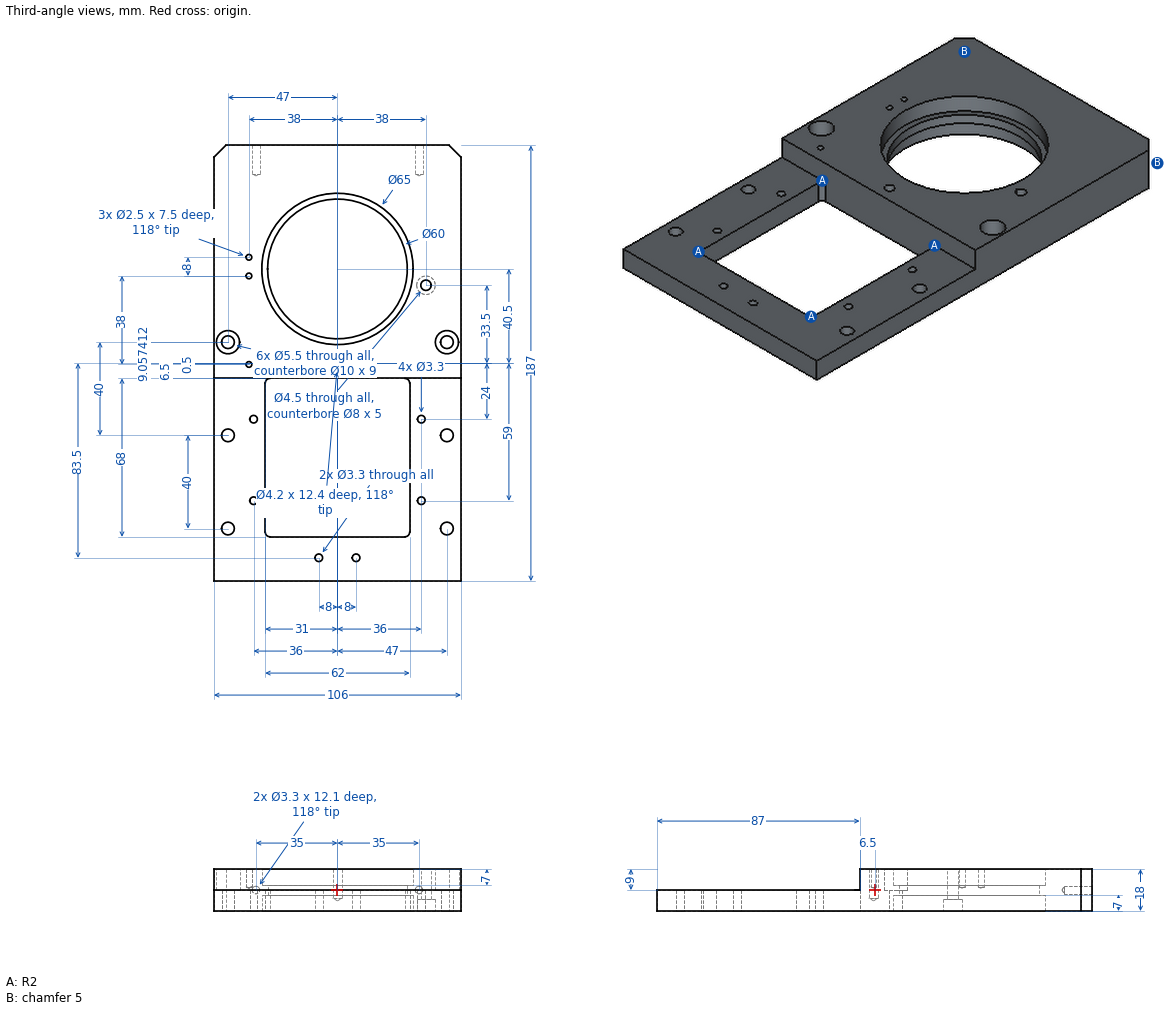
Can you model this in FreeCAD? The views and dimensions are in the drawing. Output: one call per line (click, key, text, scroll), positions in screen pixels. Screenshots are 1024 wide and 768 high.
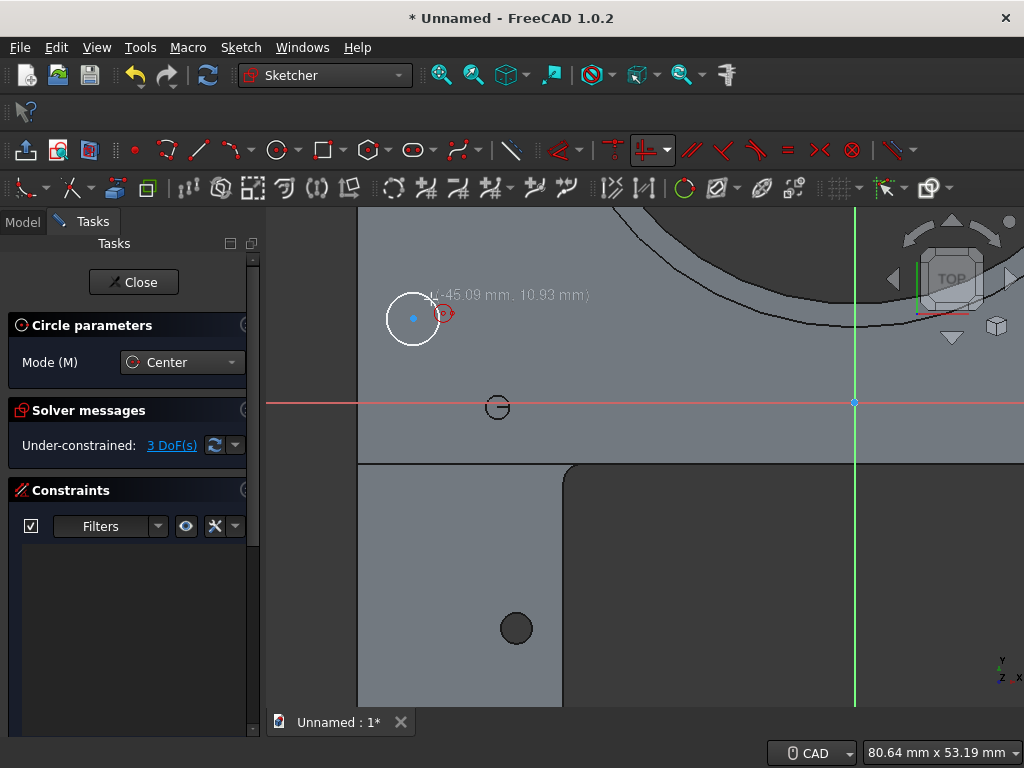
scroll(415, 319, down, 5)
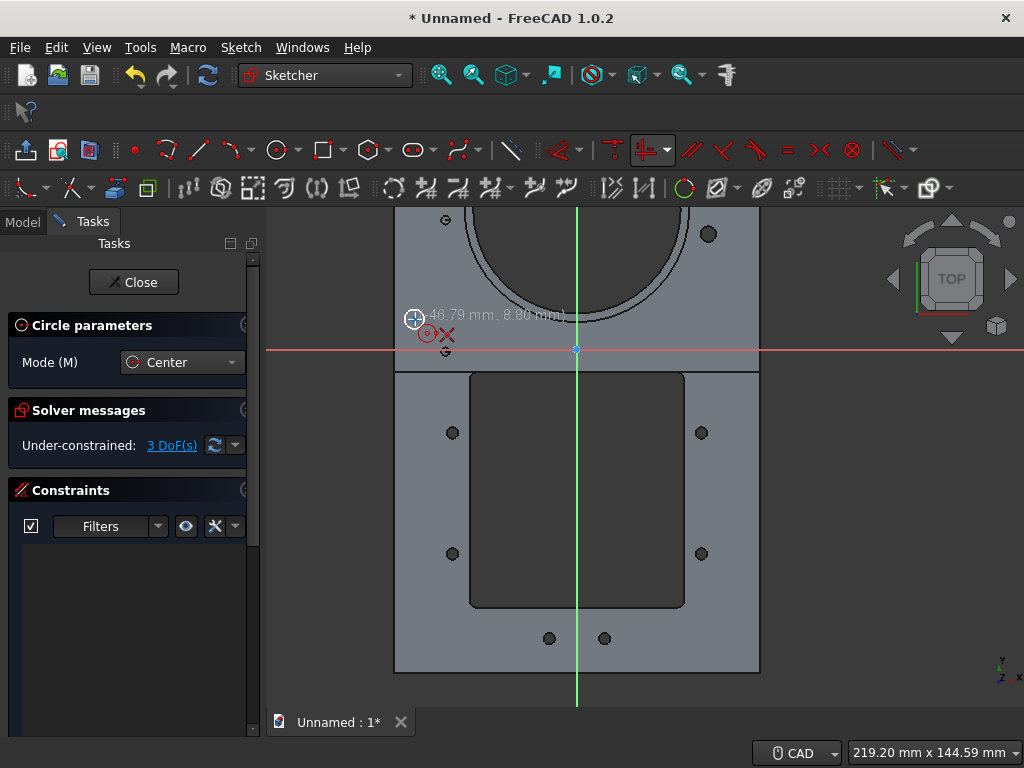
scroll(414, 457, up, 5)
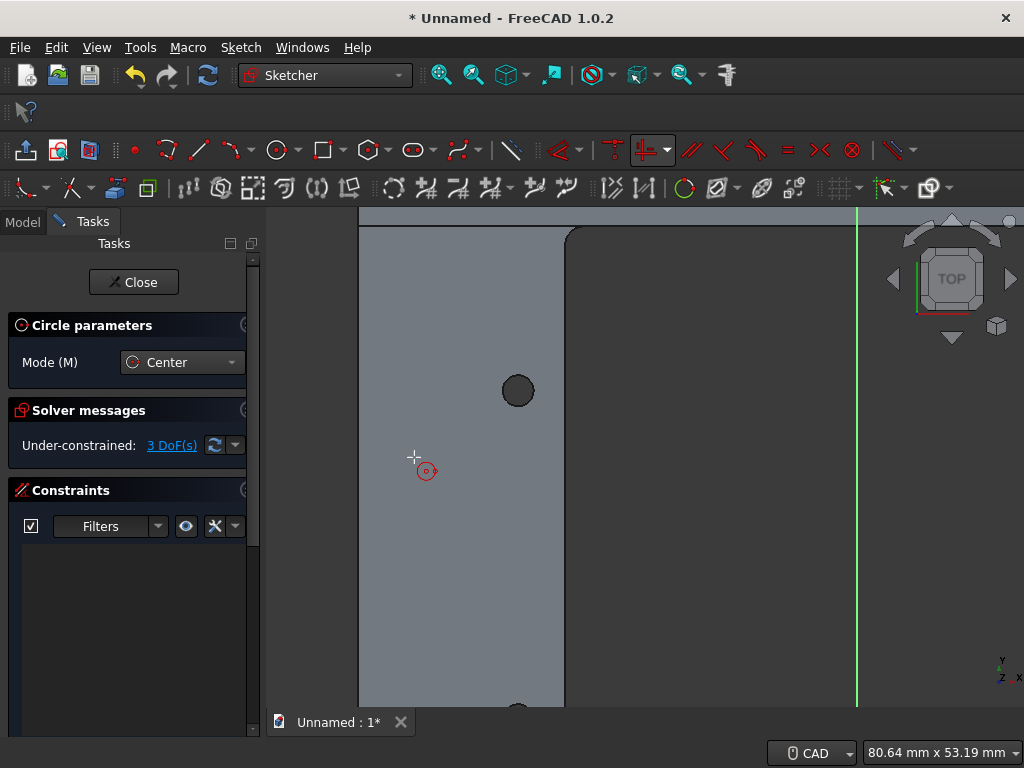
click(415, 456)
click(433, 438)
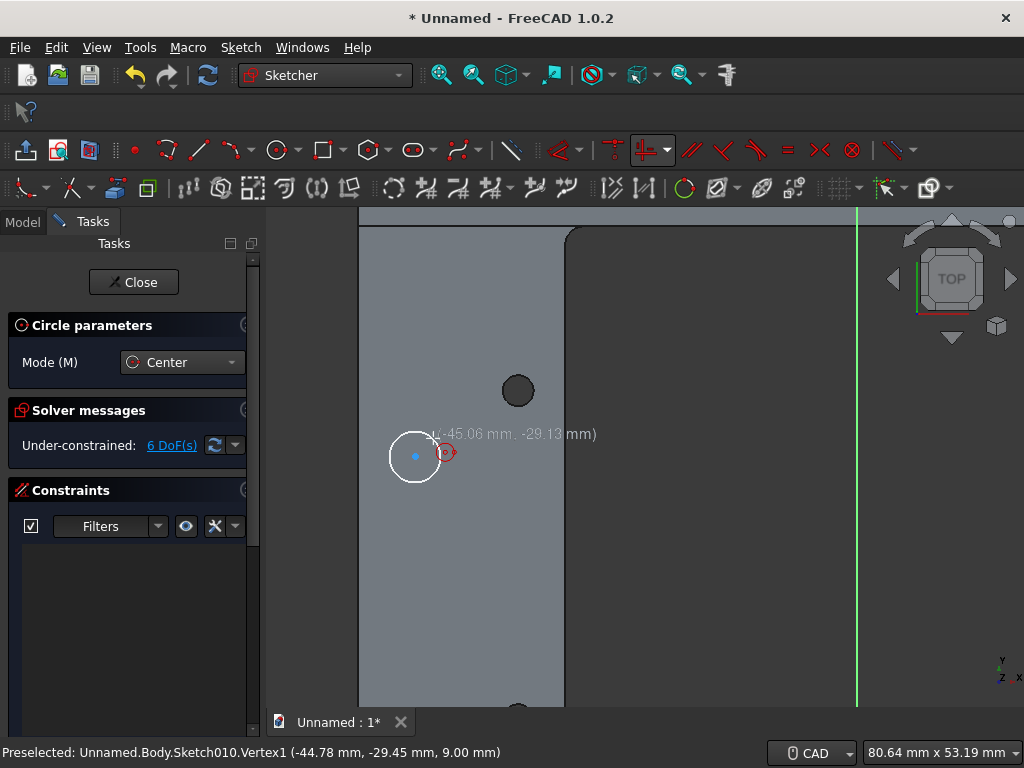
scroll(414, 458, down, 5)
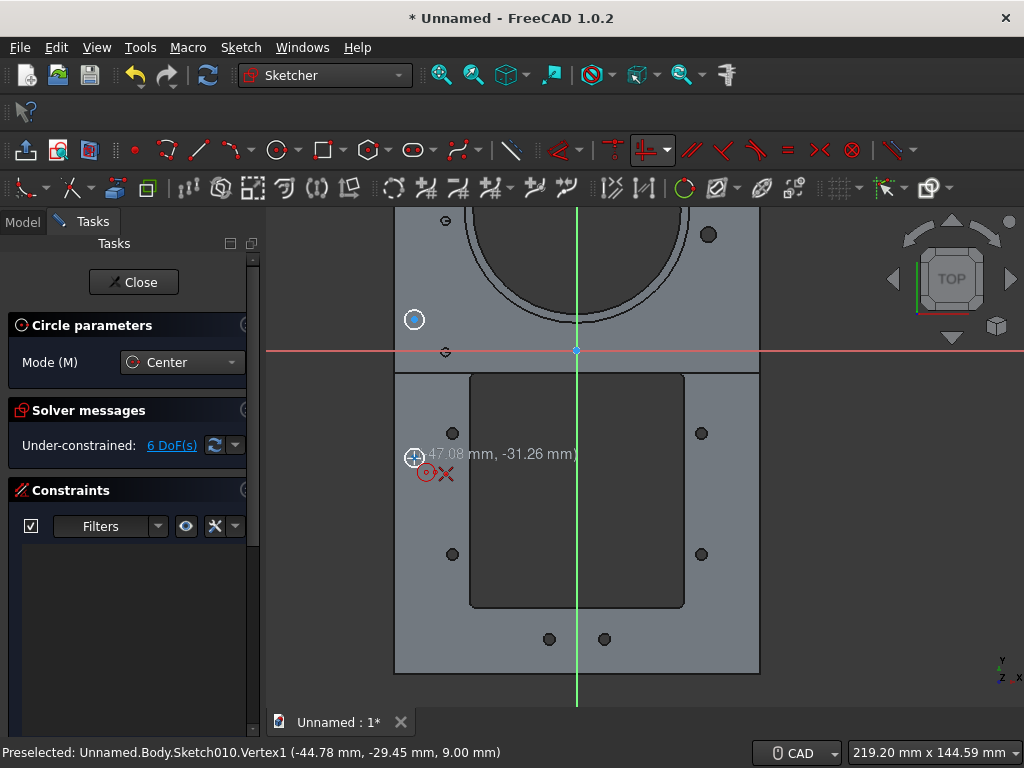
scroll(414, 596, up, 5)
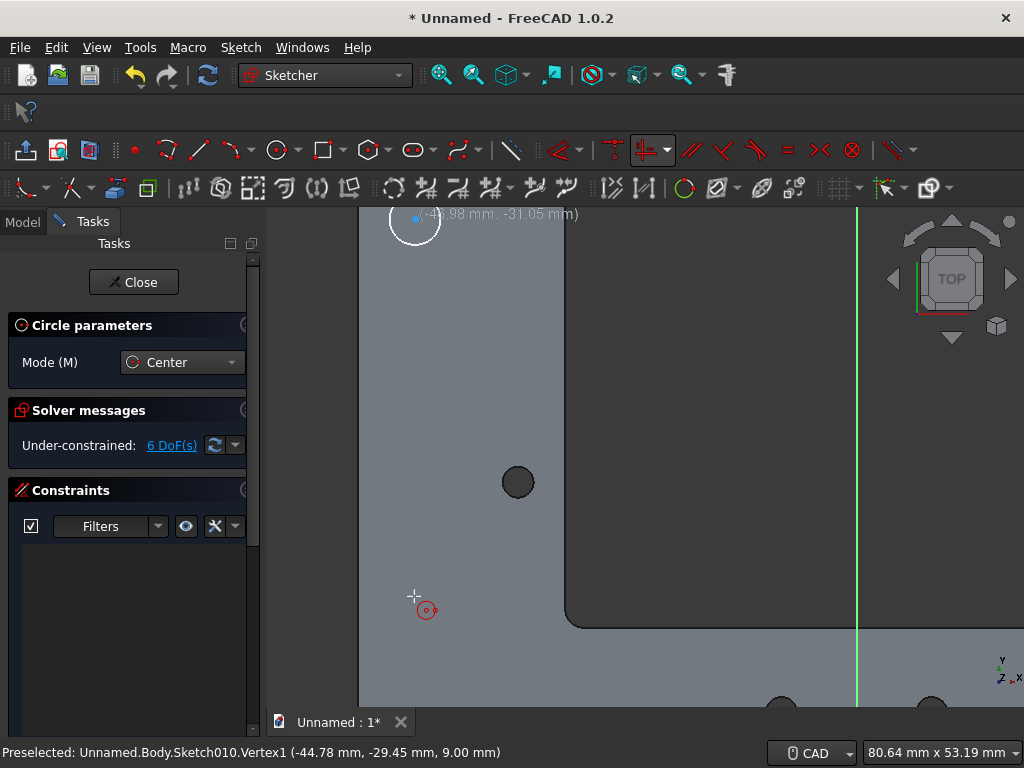
click(415, 594)
click(433, 576)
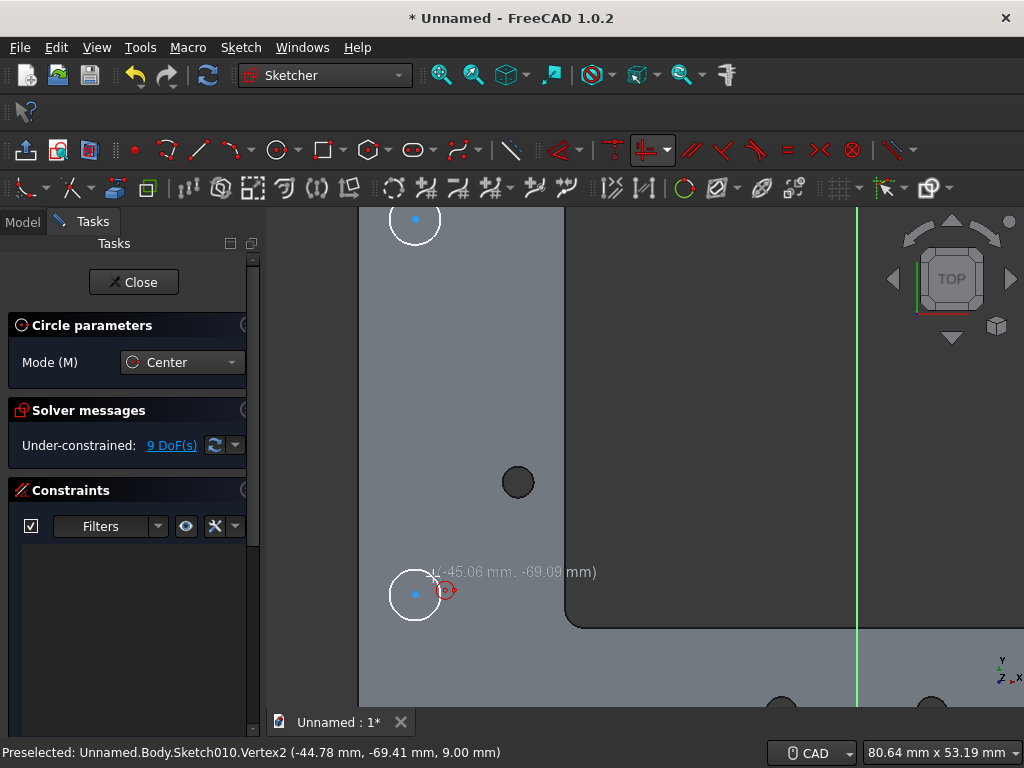
scroll(414, 596, down, 5)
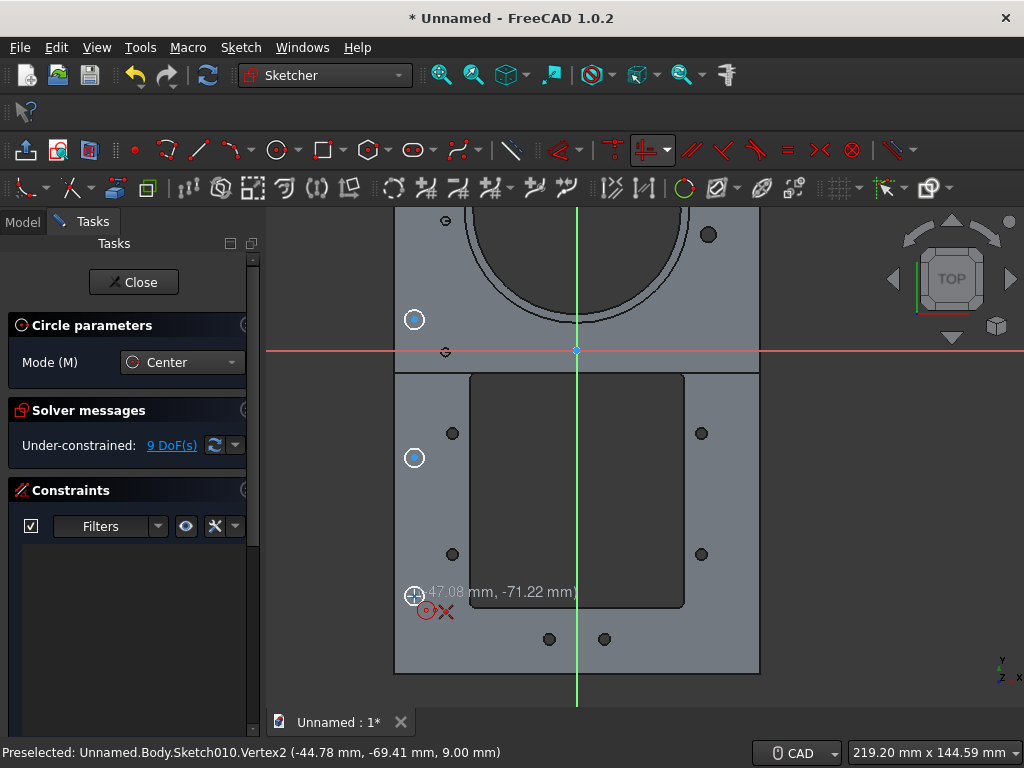
scroll(739, 596, up, 5)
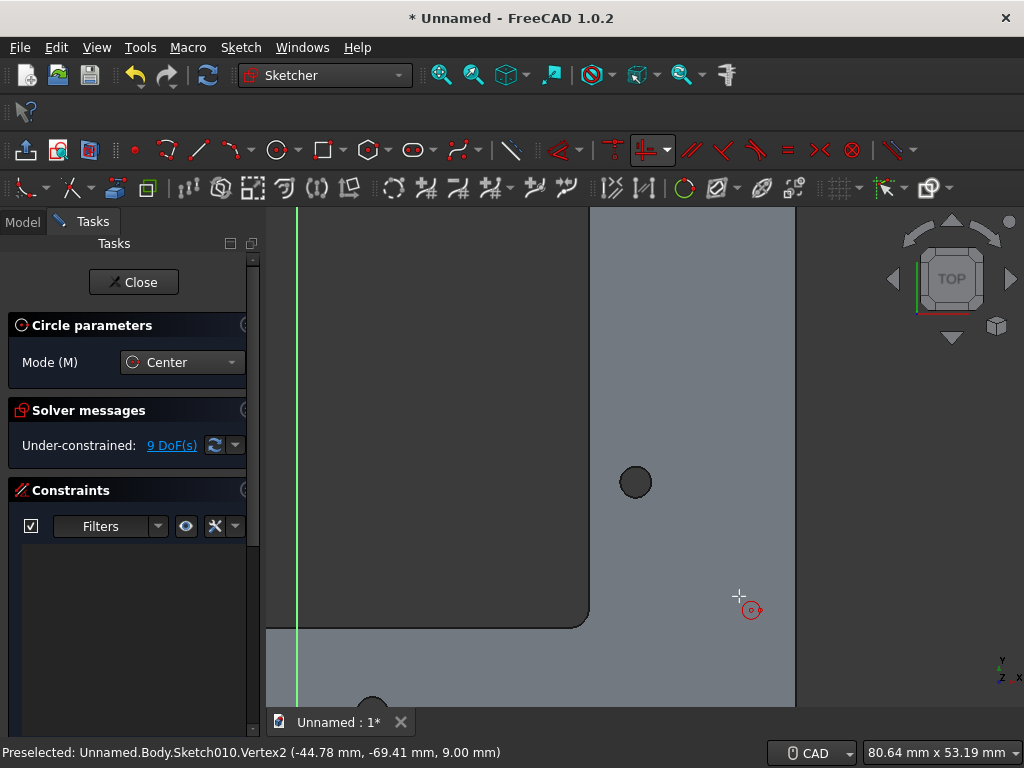
click(739, 594)
click(757, 576)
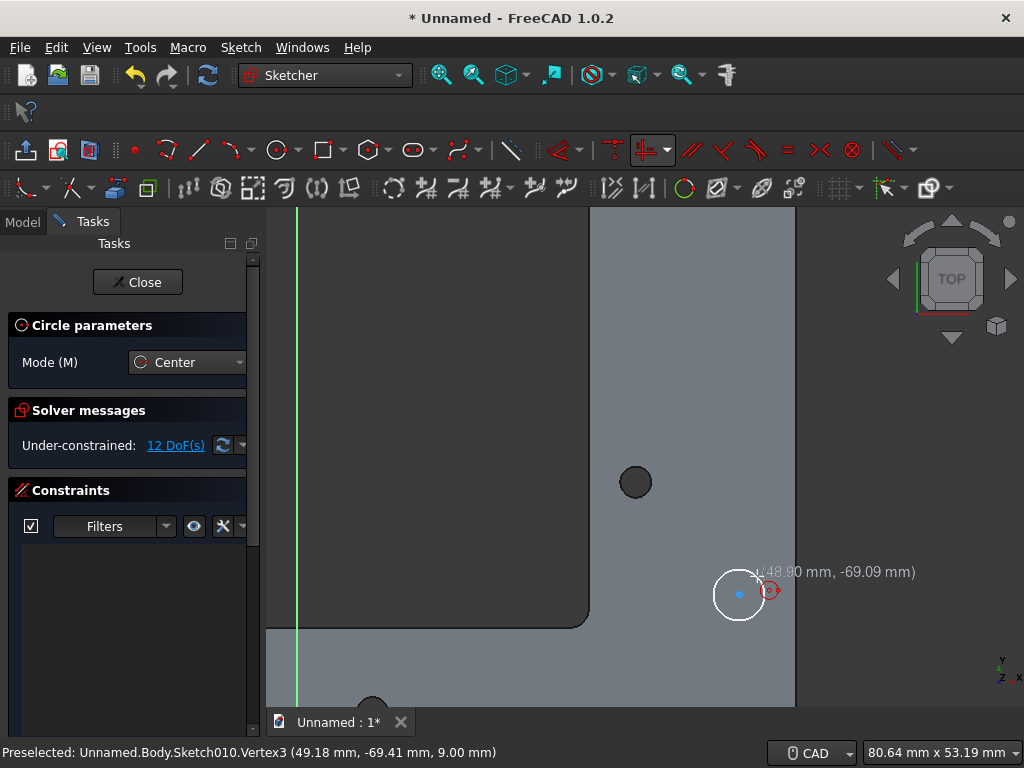
scroll(739, 596, down, 5)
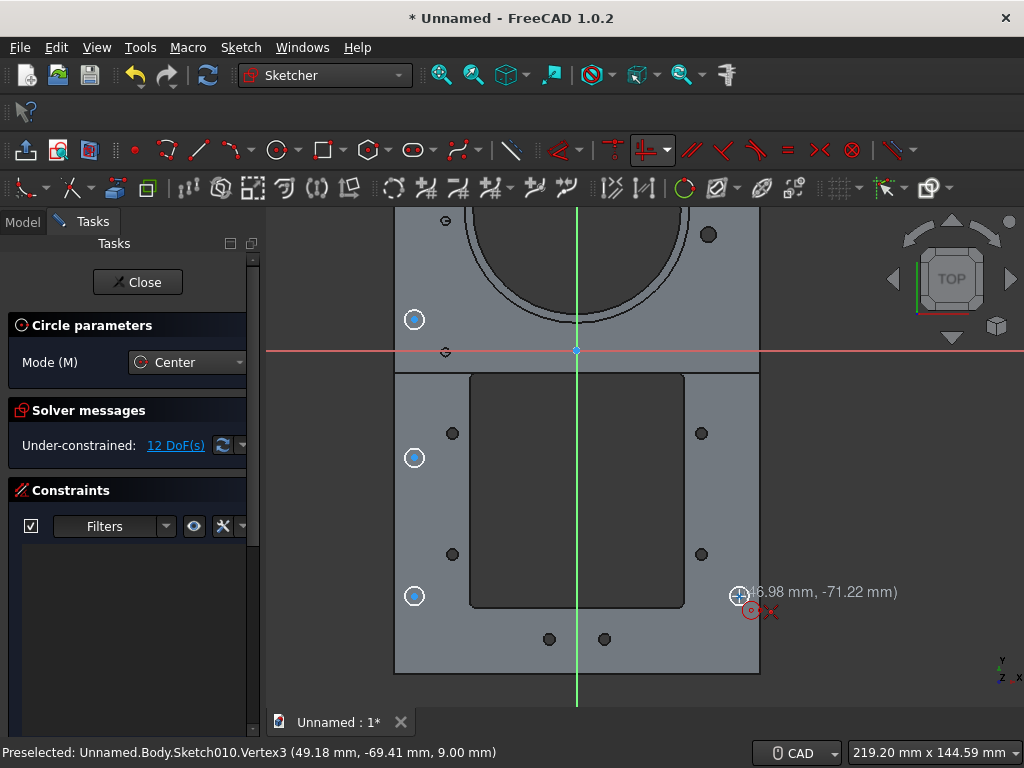
scroll(739, 458, up, 5)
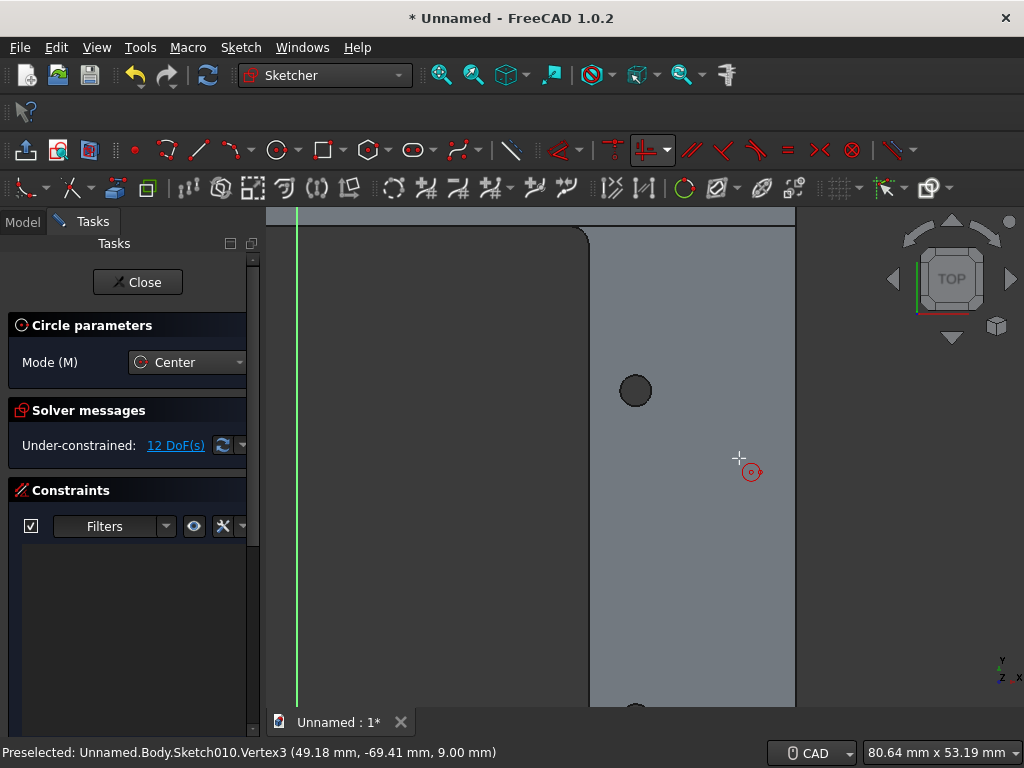
click(739, 456)
click(757, 438)